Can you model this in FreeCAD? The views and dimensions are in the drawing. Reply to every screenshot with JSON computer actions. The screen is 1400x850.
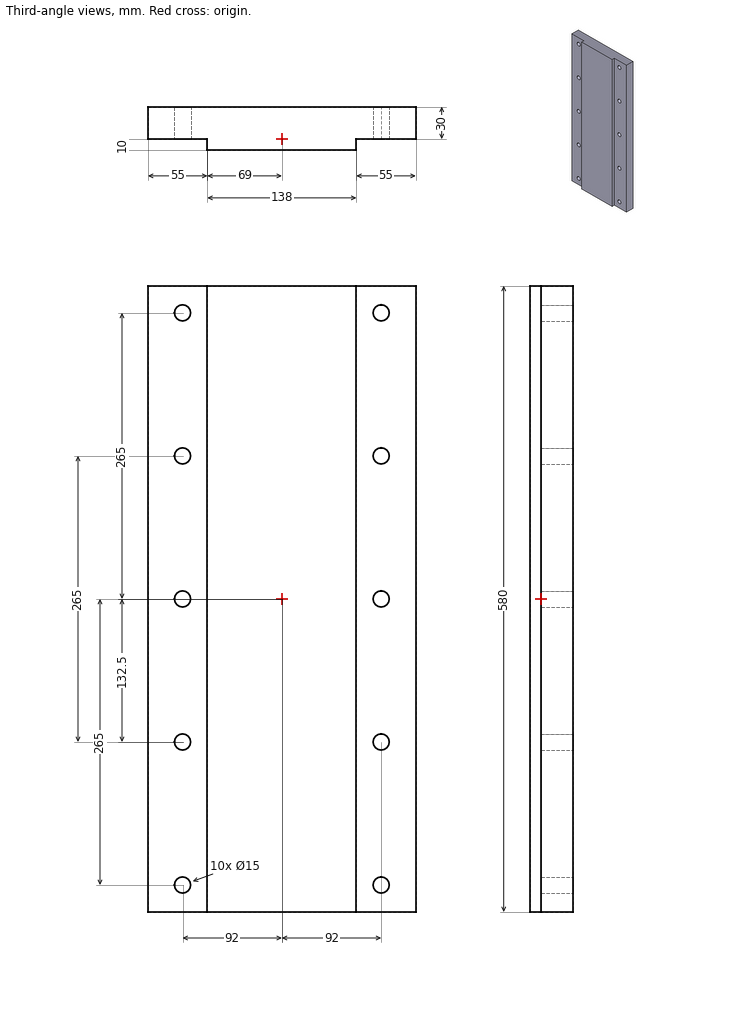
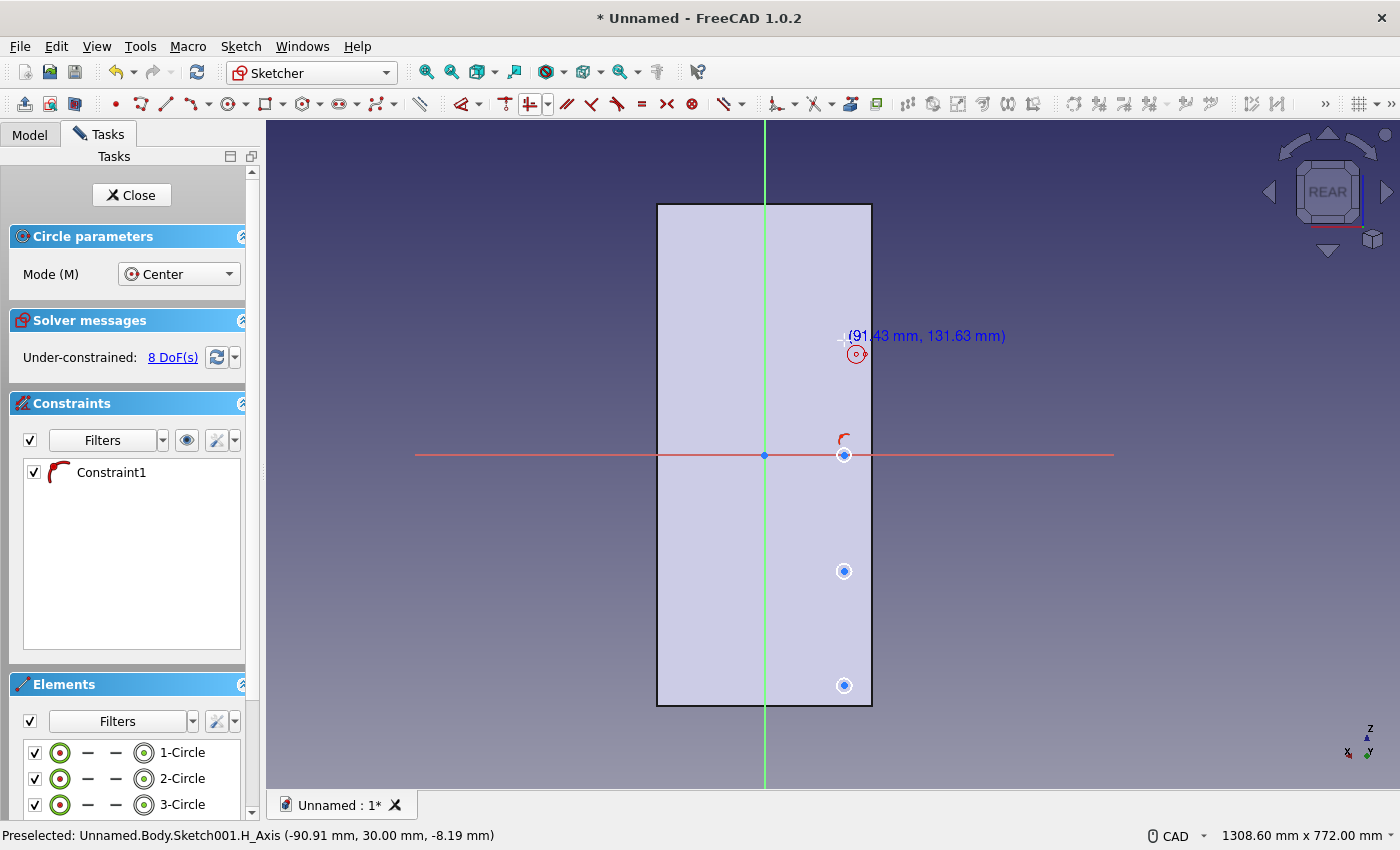
{"action": "left_click", "coordinate": [844, 340]}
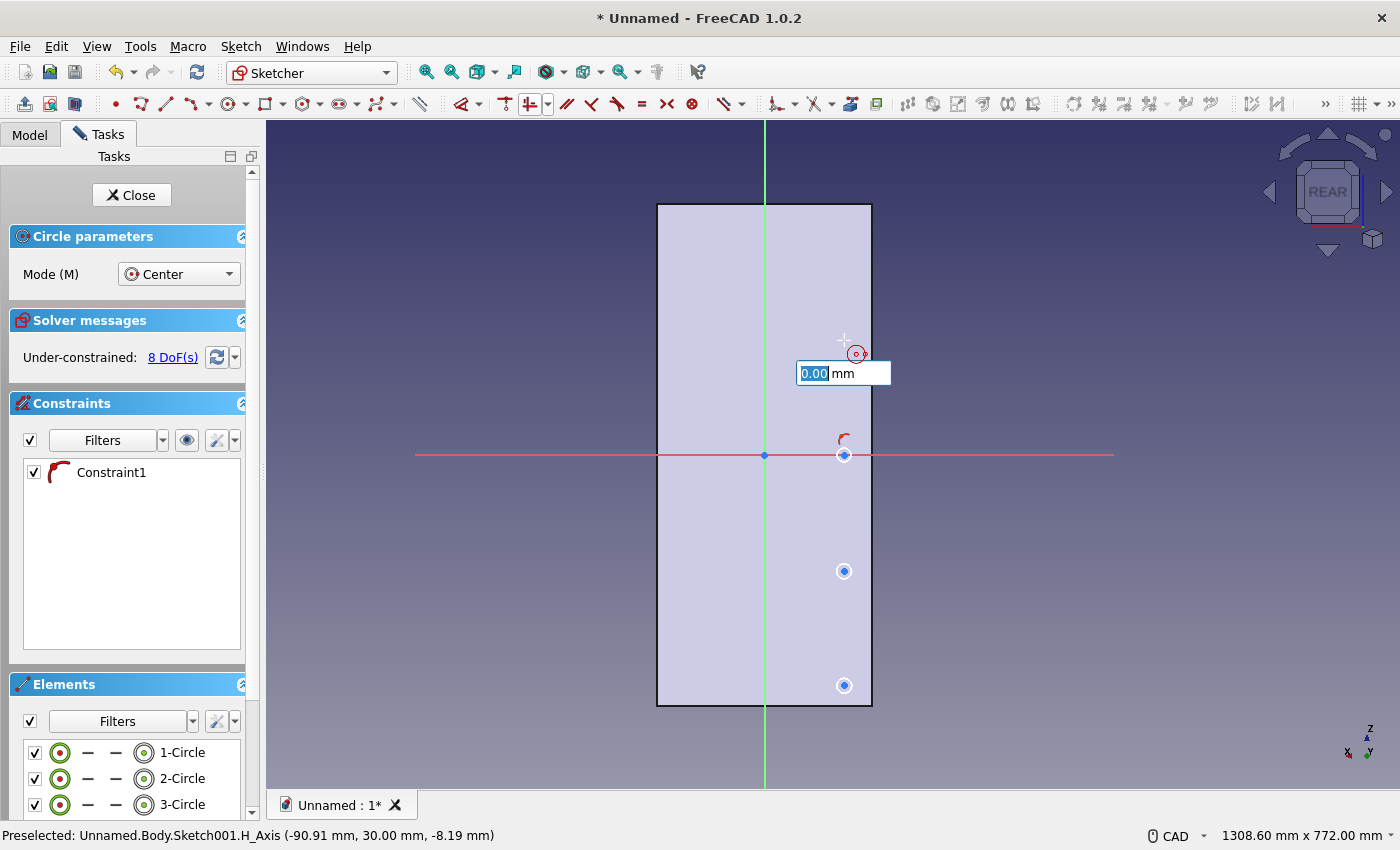
{"action": "scroll", "coordinate": [849, 336], "scroll_direction": "up", "scroll_amount": 5}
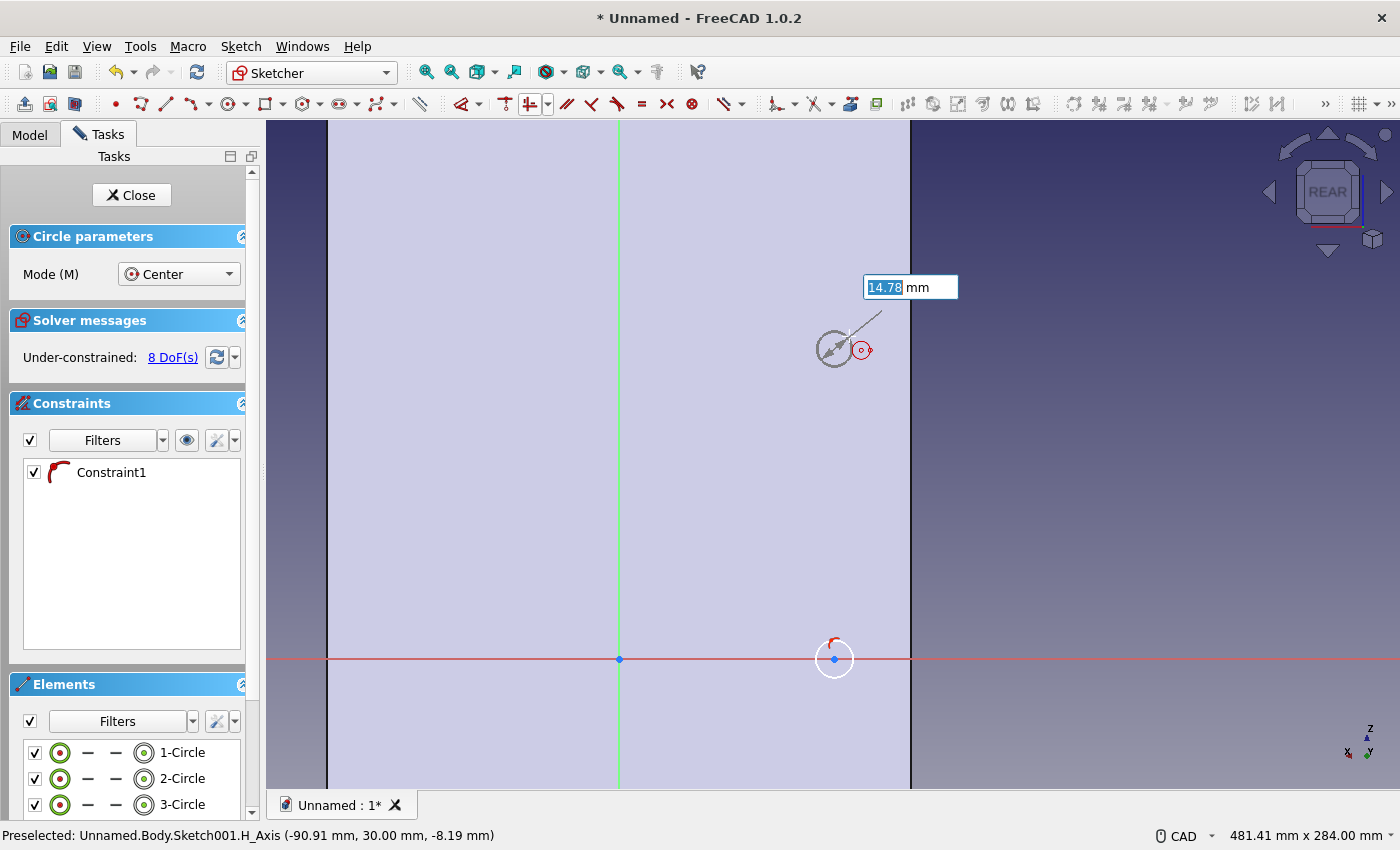
{"action": "left_click", "coordinate": [848, 334]}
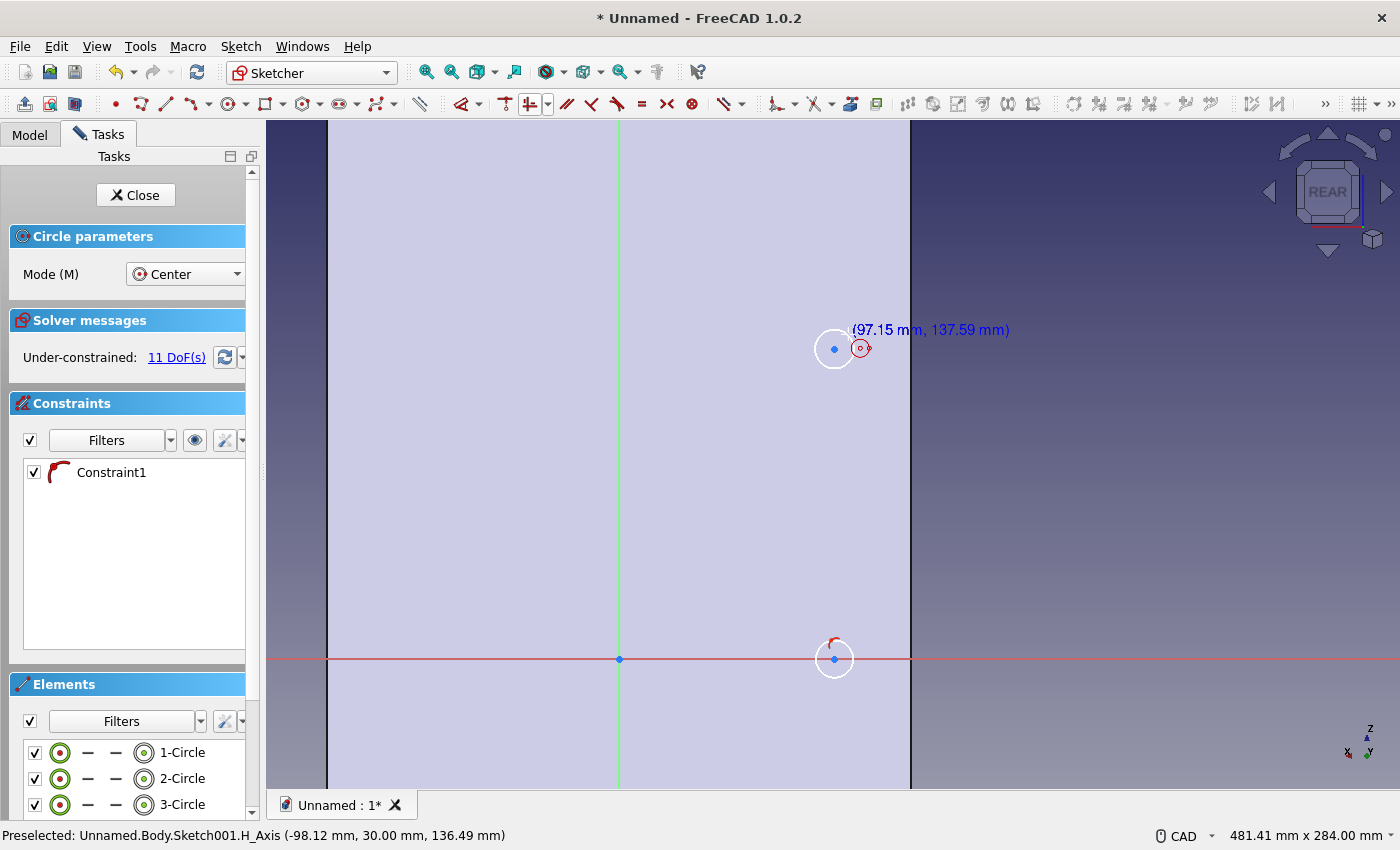
{"action": "scroll", "coordinate": [849, 335], "scroll_direction": "down", "scroll_amount": 5}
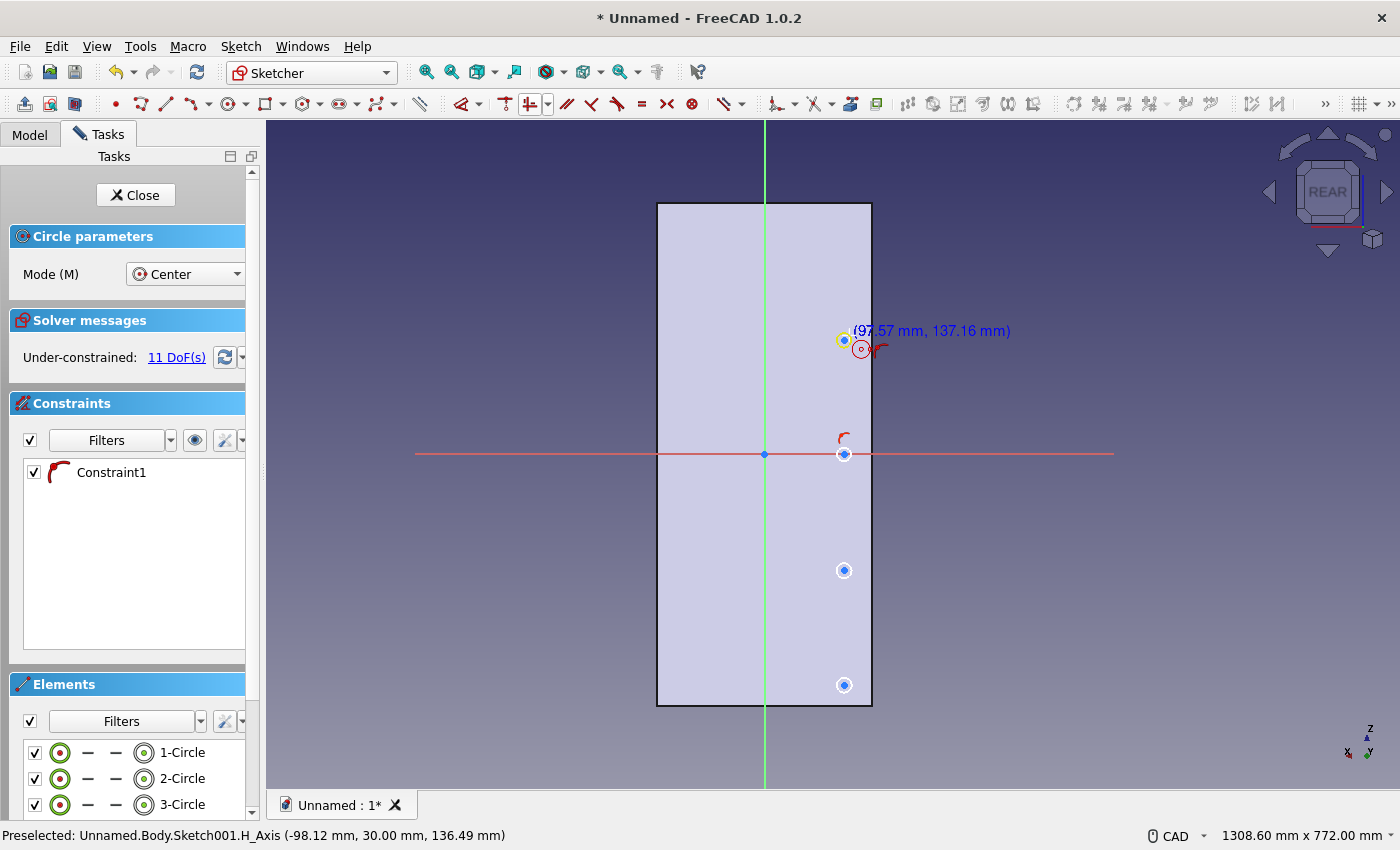
{"action": "scroll", "coordinate": [844, 225], "scroll_direction": "up", "scroll_amount": 7}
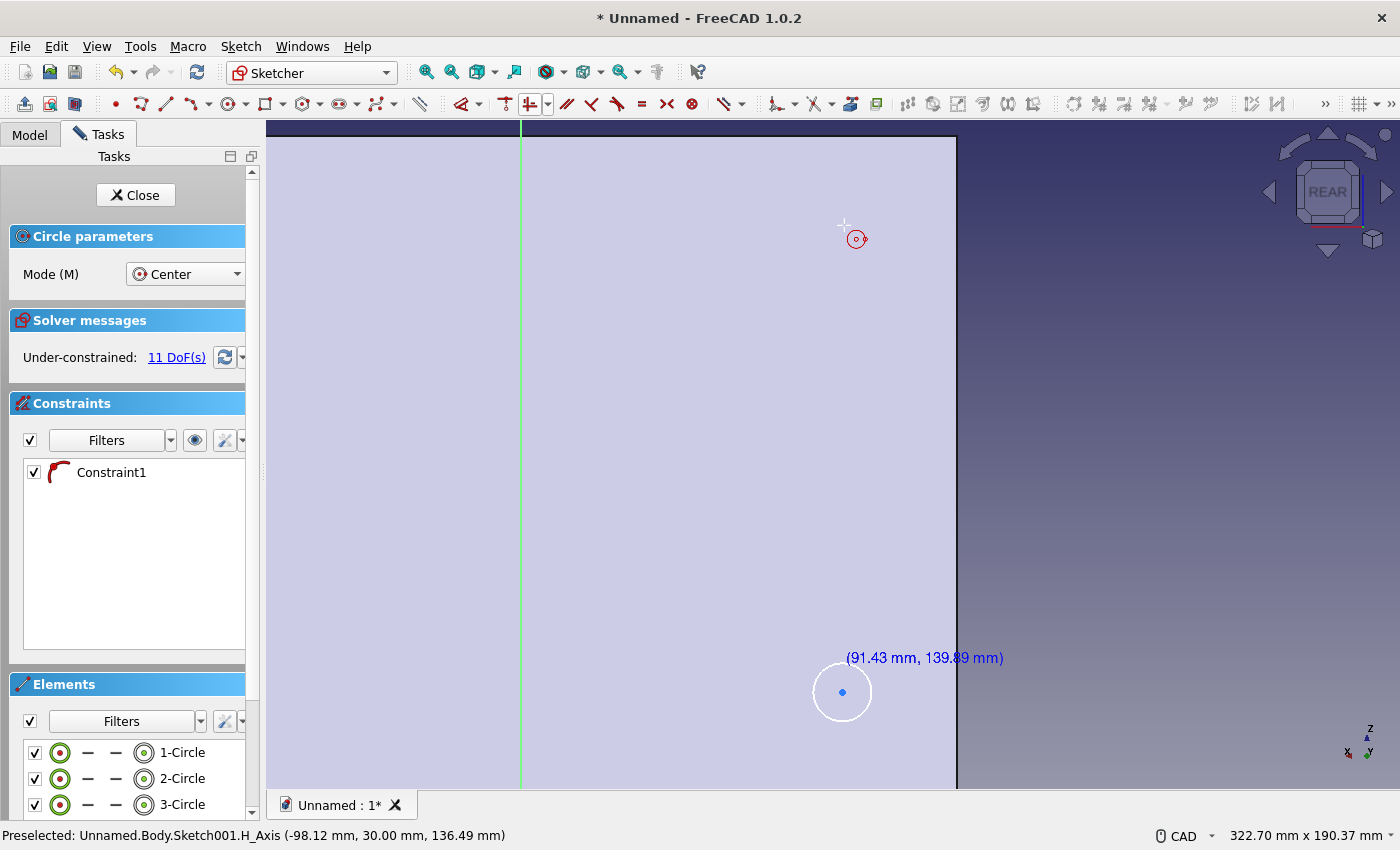
{"action": "scroll", "coordinate": [844, 225], "scroll_direction": "down", "scroll_amount": 7}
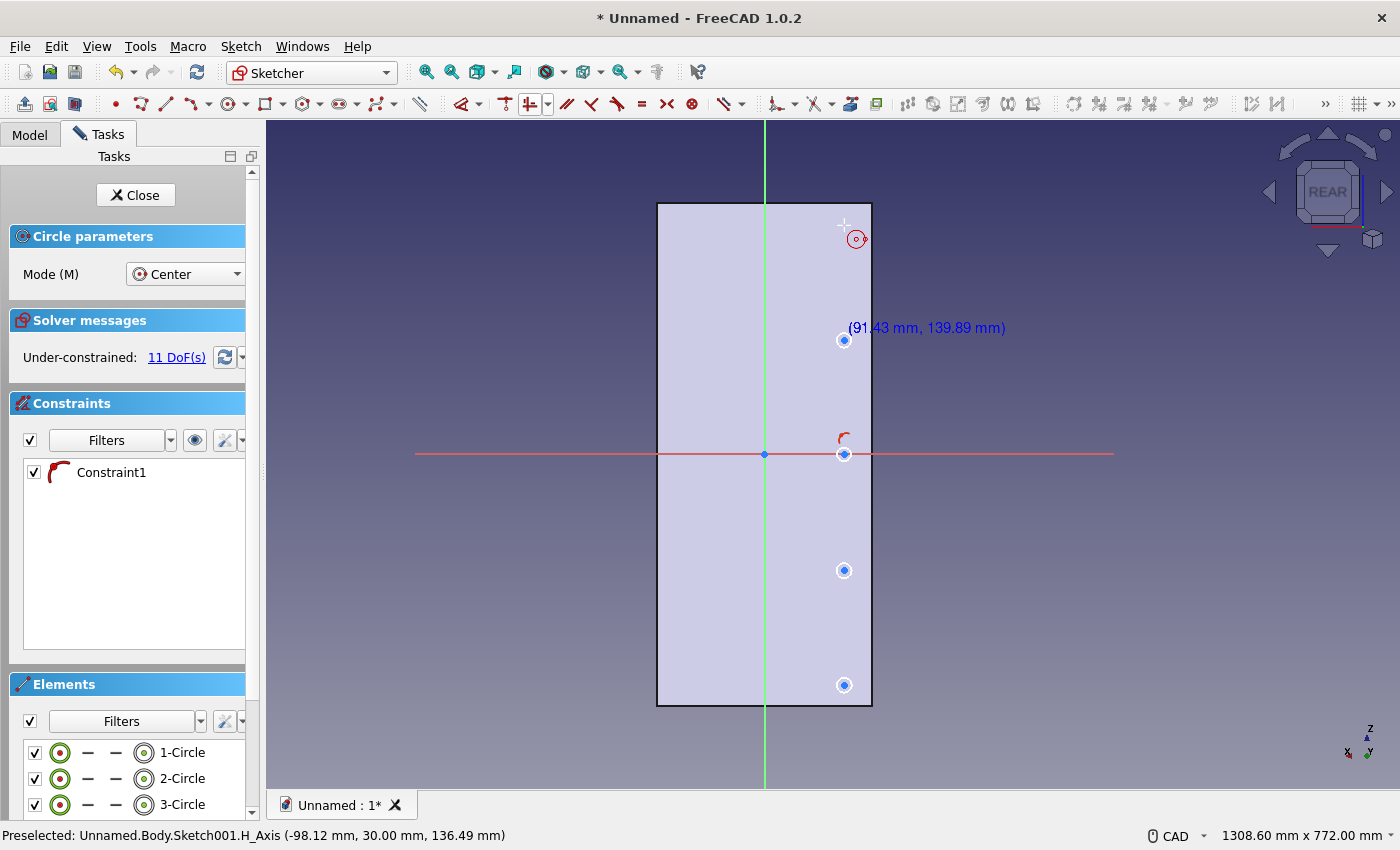
{"action": "left_click", "coordinate": [844, 225]}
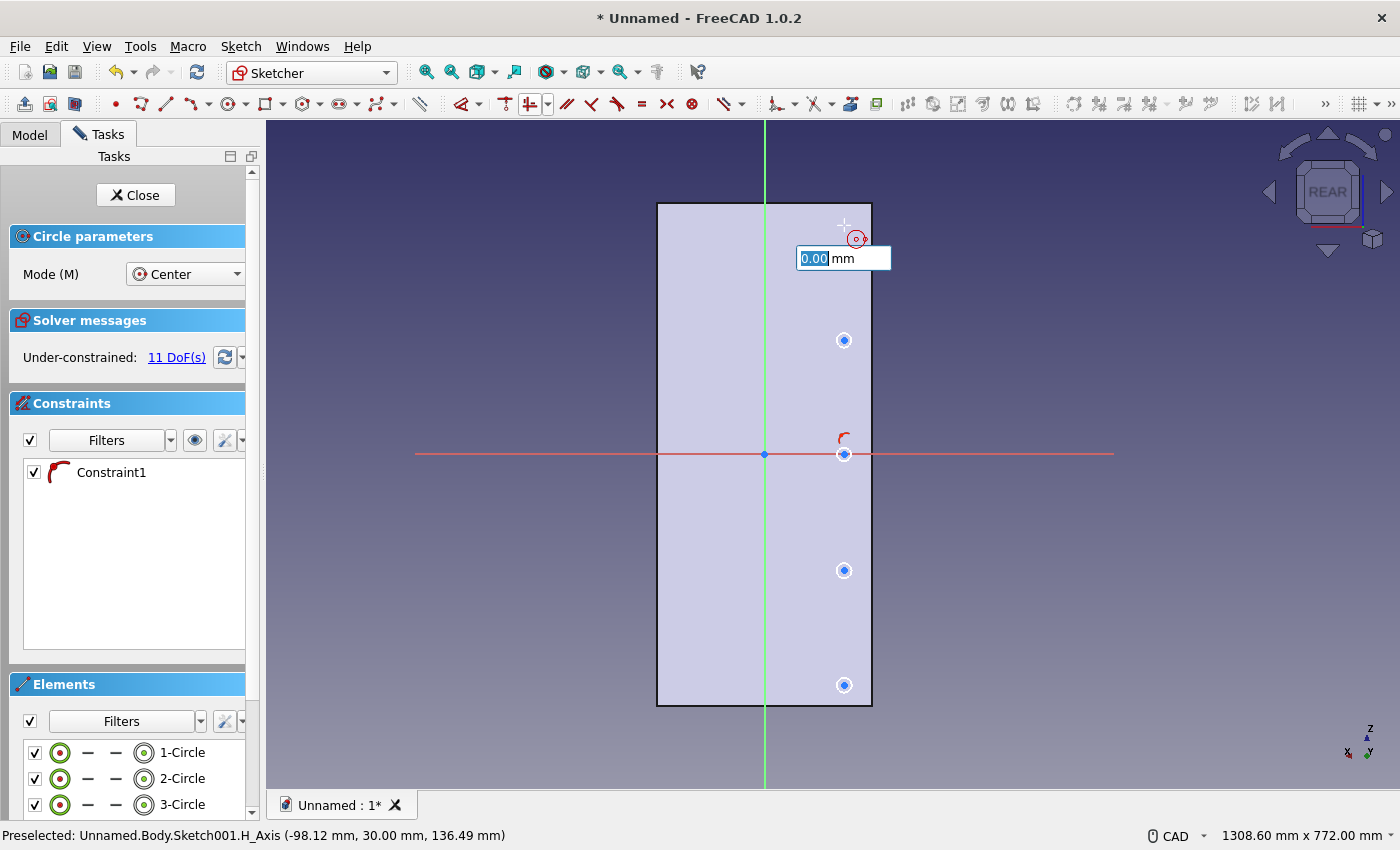
{"action": "scroll", "coordinate": [849, 220], "scroll_direction": "up", "scroll_amount": 5}